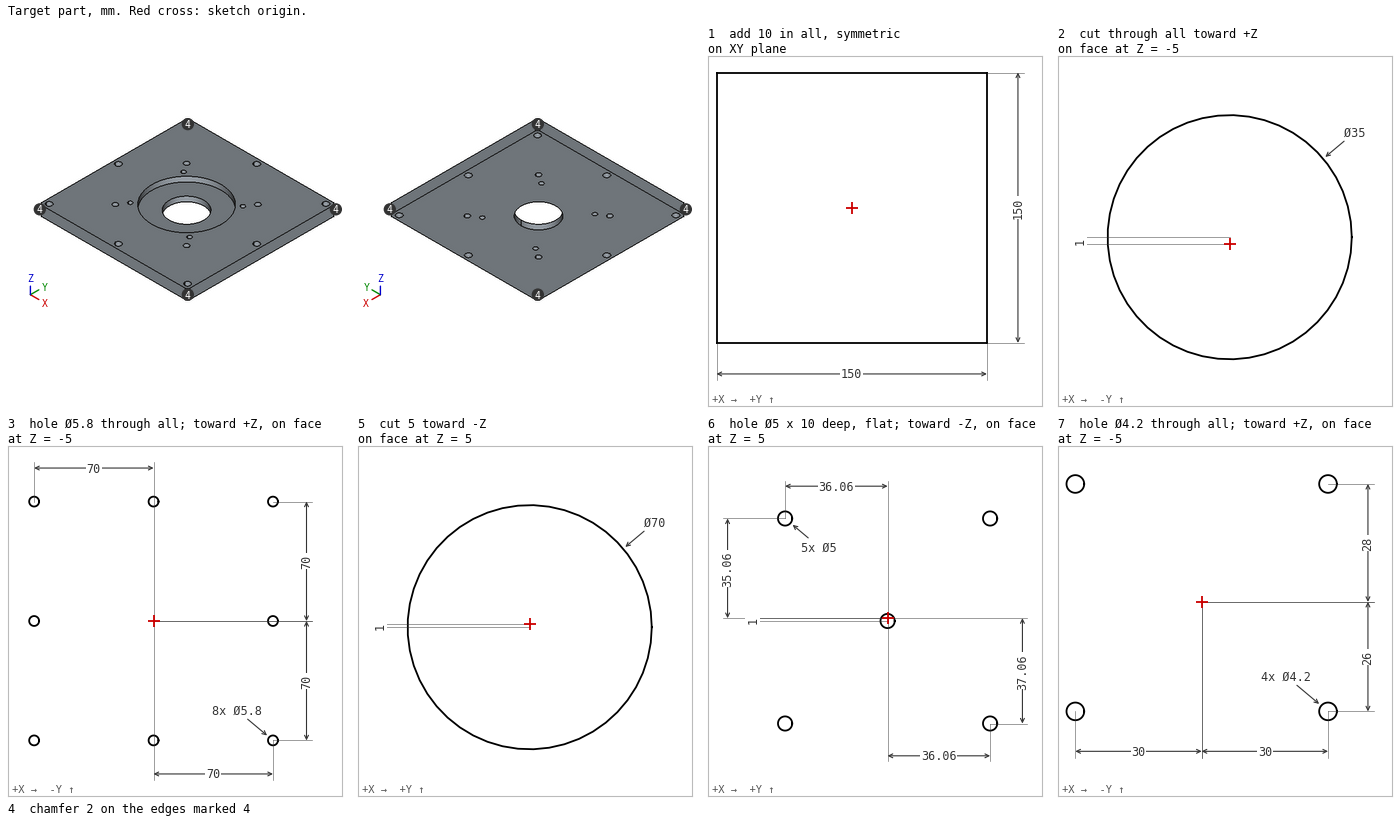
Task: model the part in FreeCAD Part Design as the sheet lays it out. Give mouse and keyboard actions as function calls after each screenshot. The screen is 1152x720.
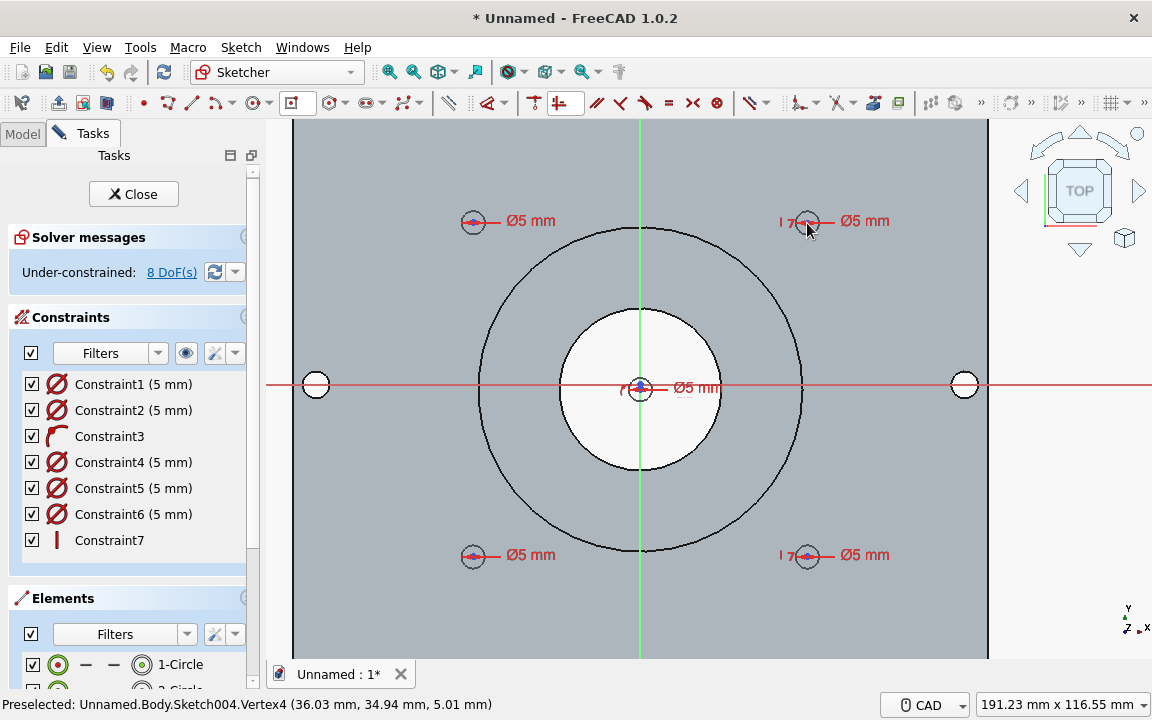
click(473, 223)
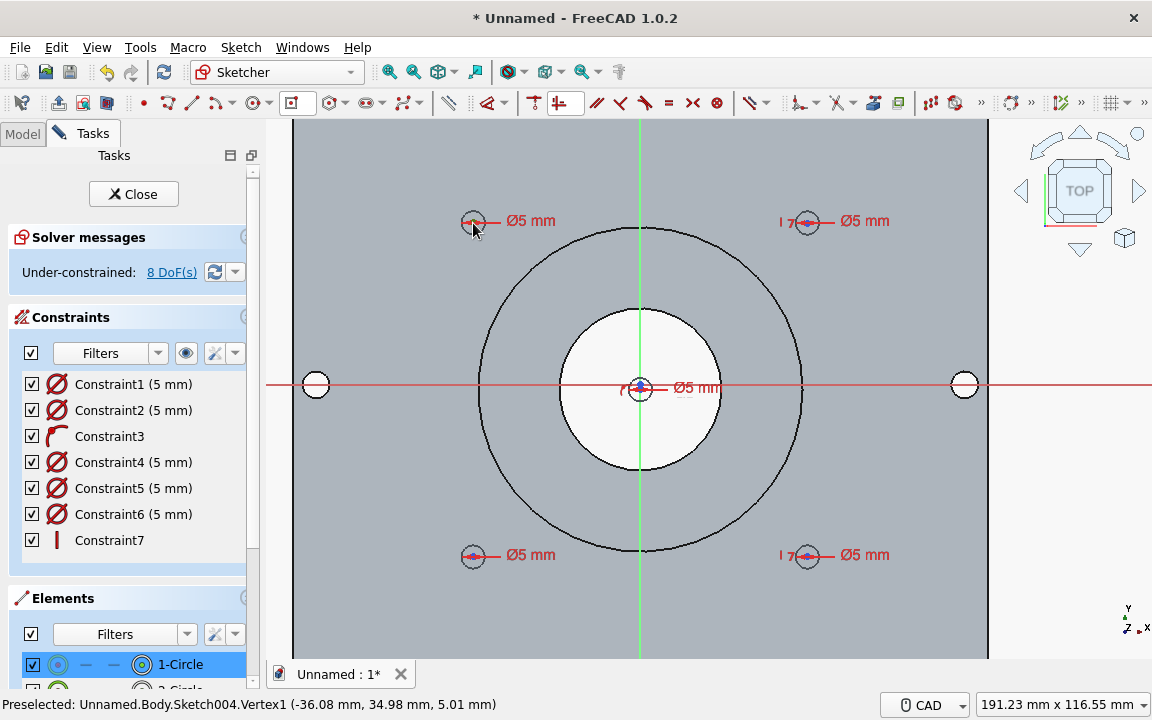
click(807, 223)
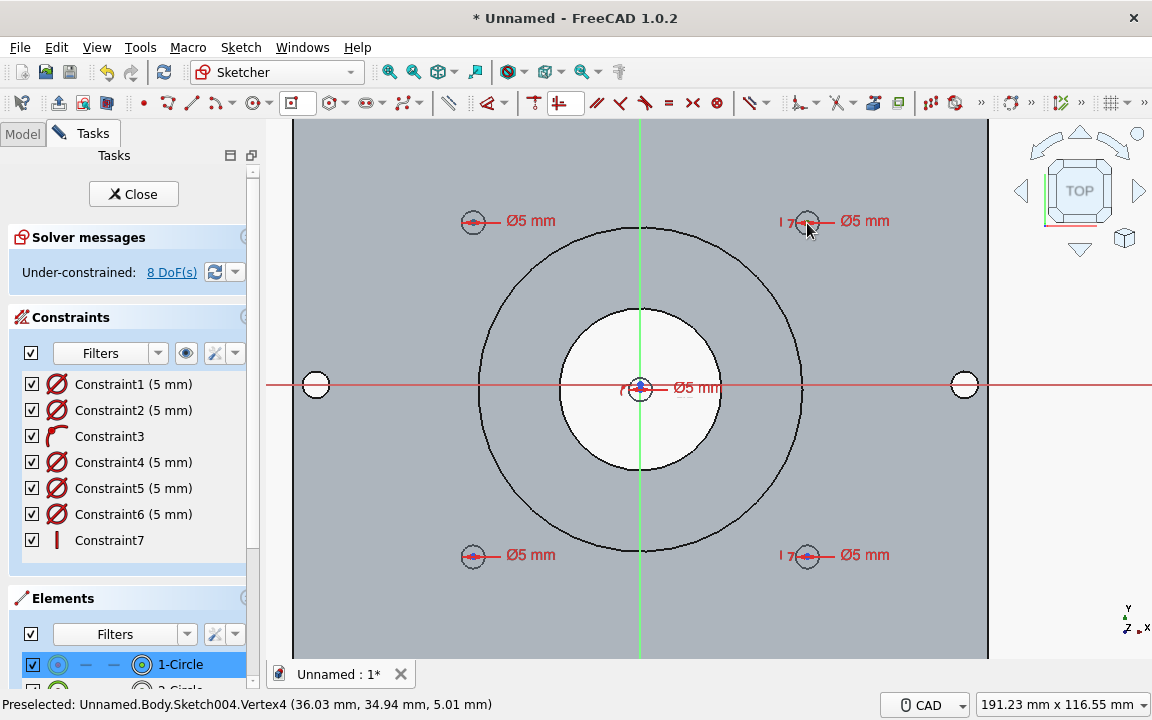
key(h)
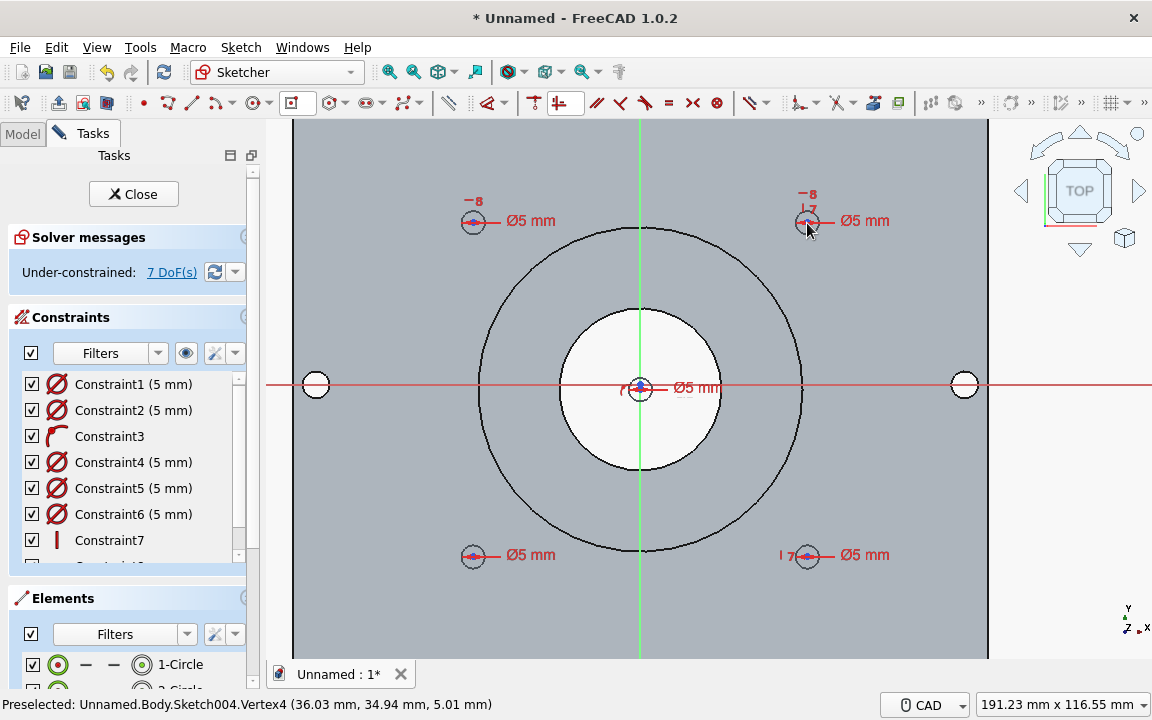
click(473, 223)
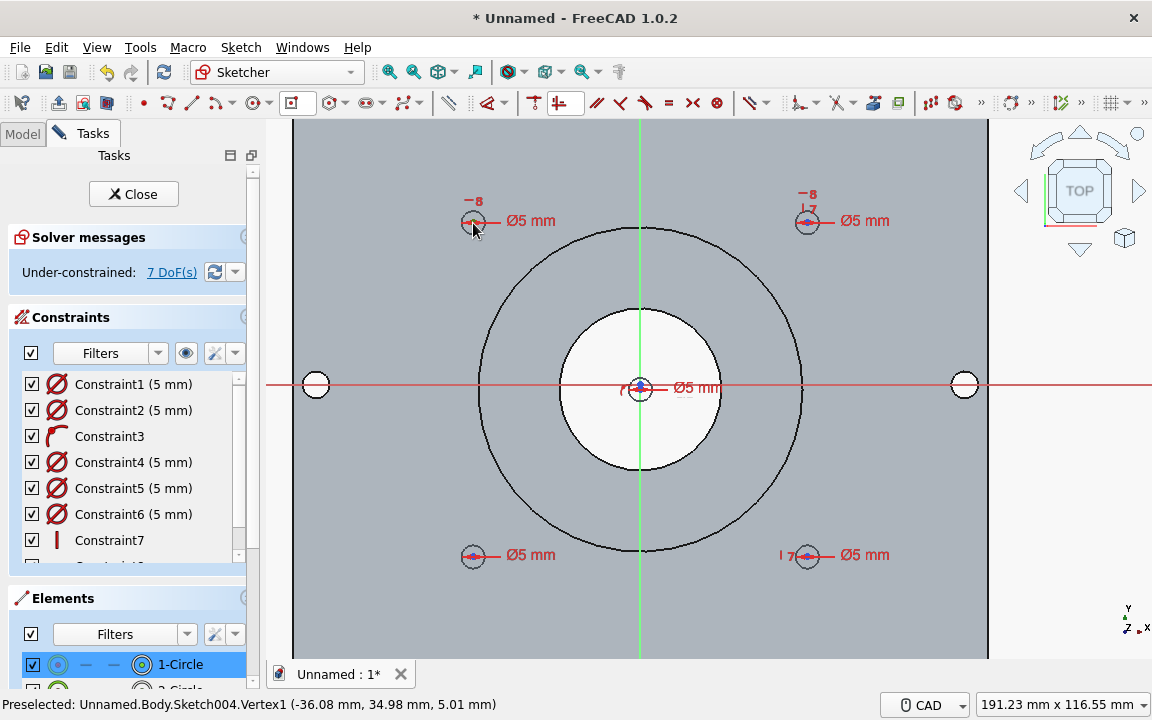
click(473, 557)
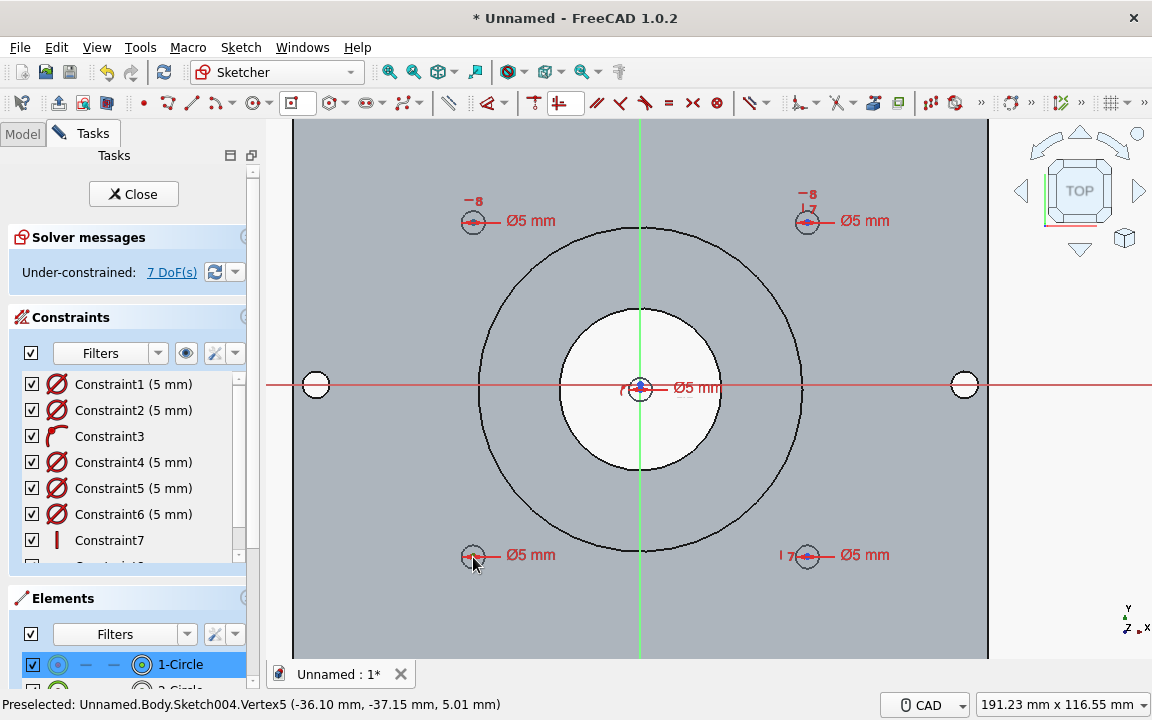
key(v)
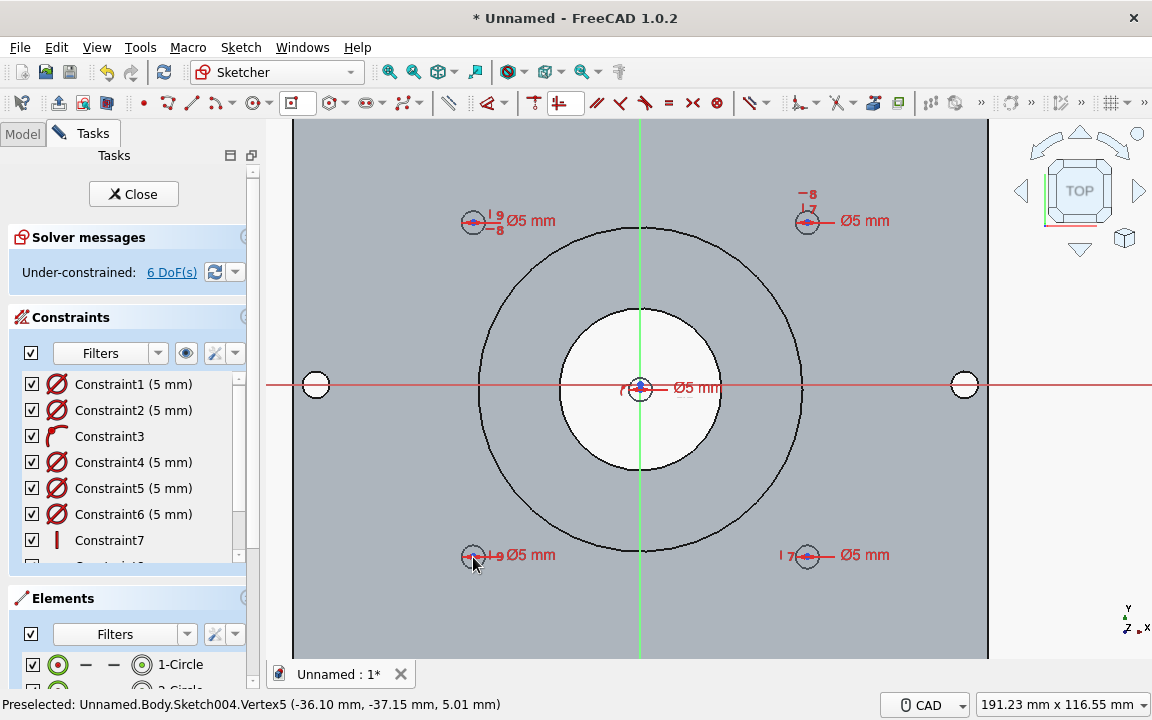
click(807, 557)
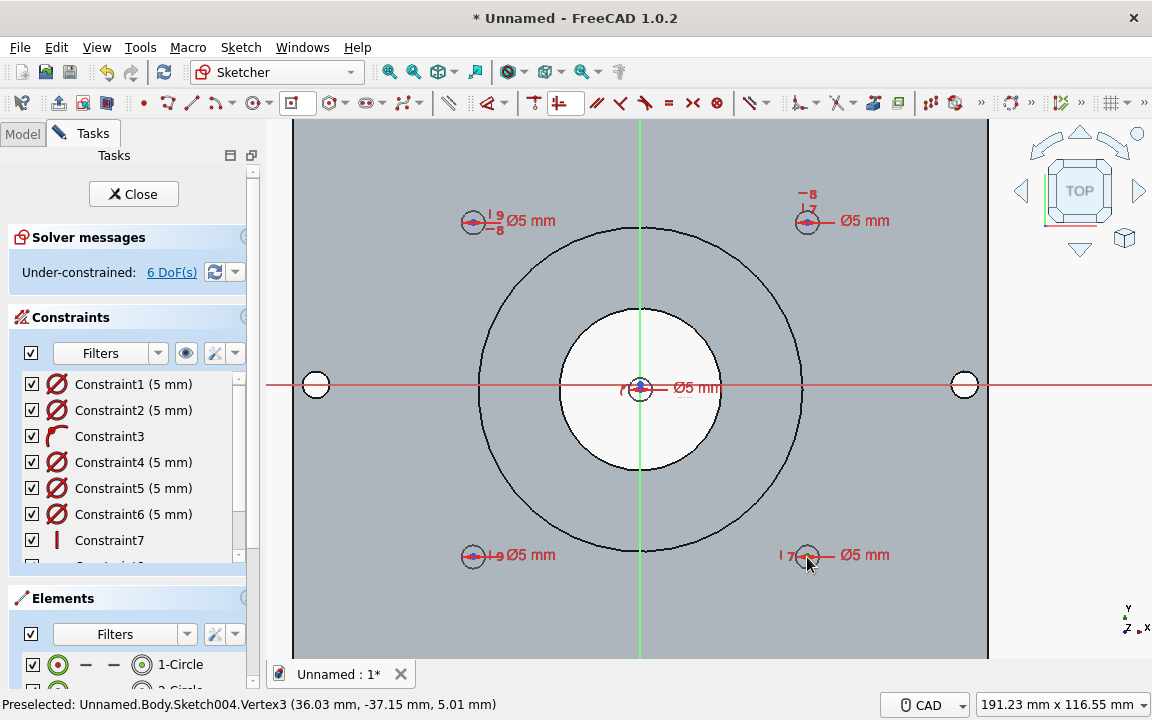
click(473, 557)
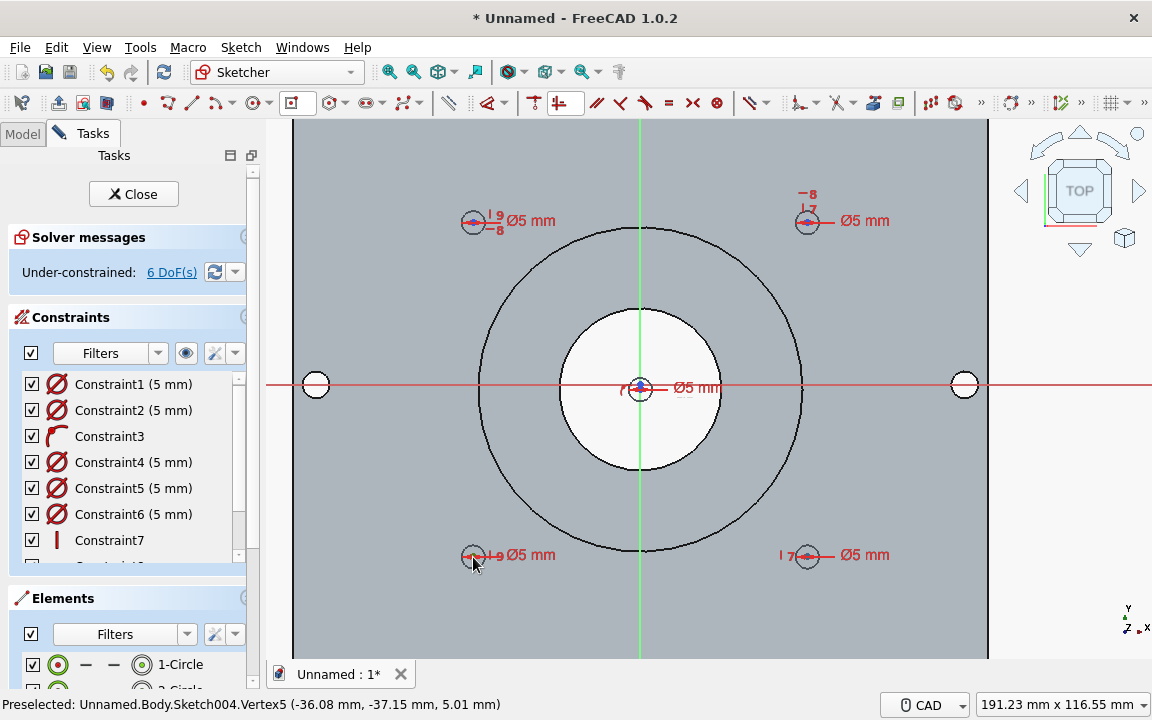
click(578, 104)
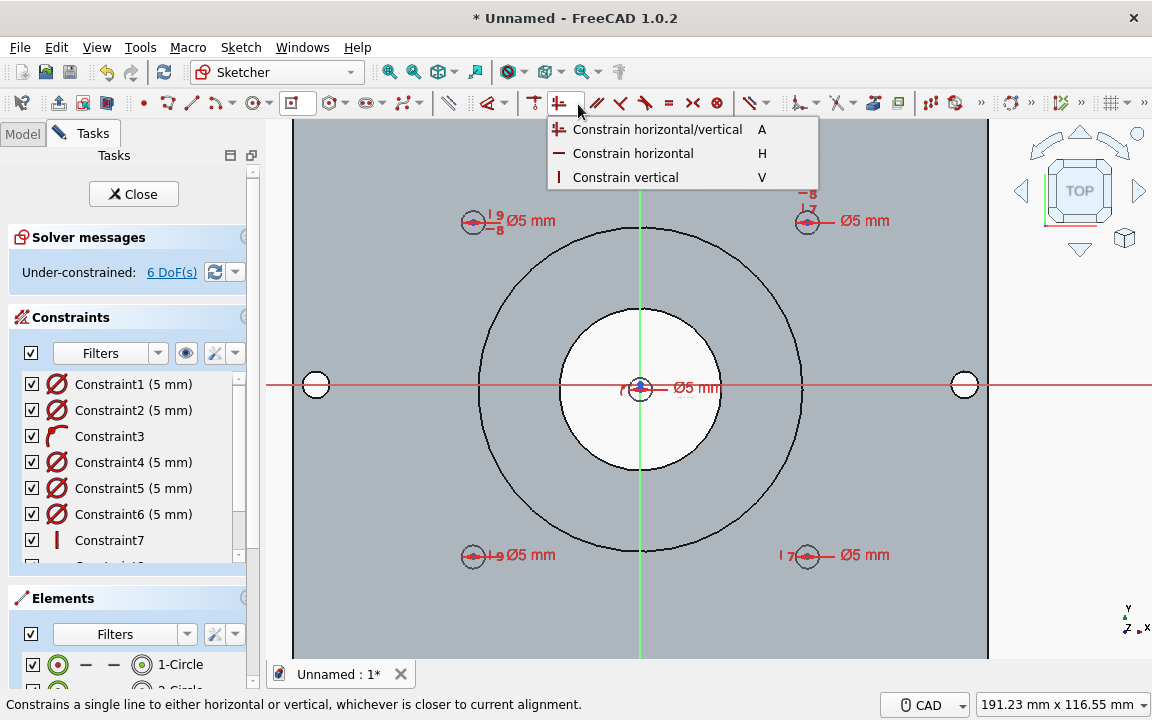
click(683, 153)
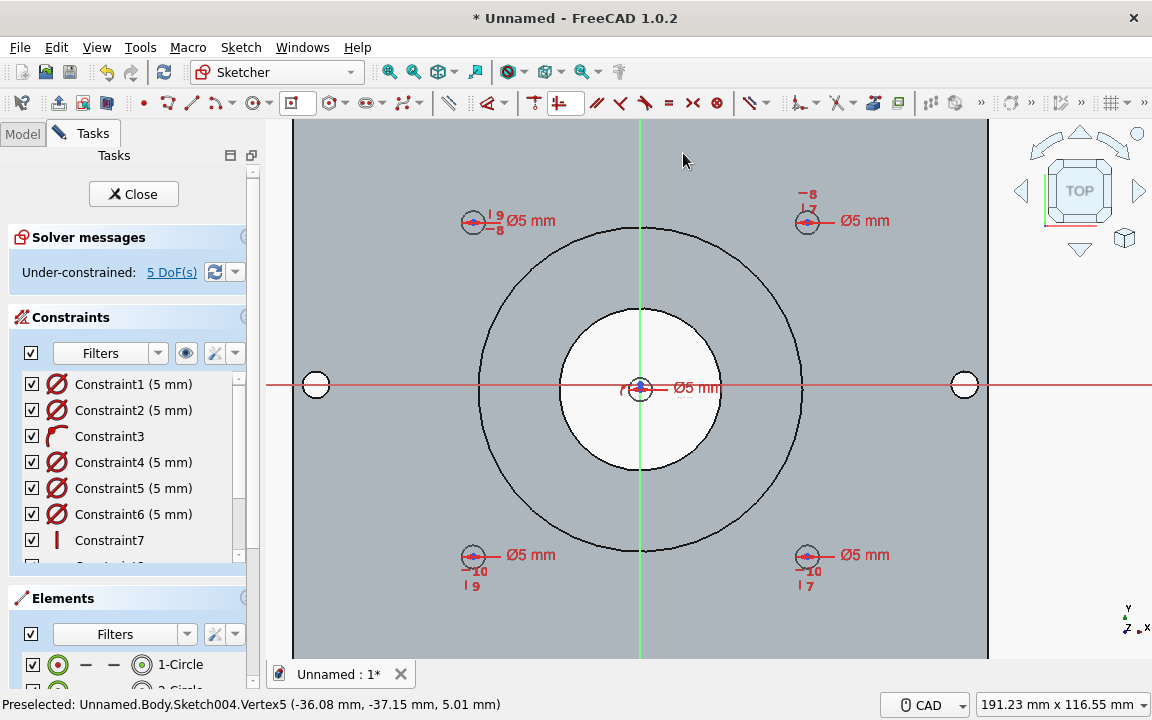
key(d)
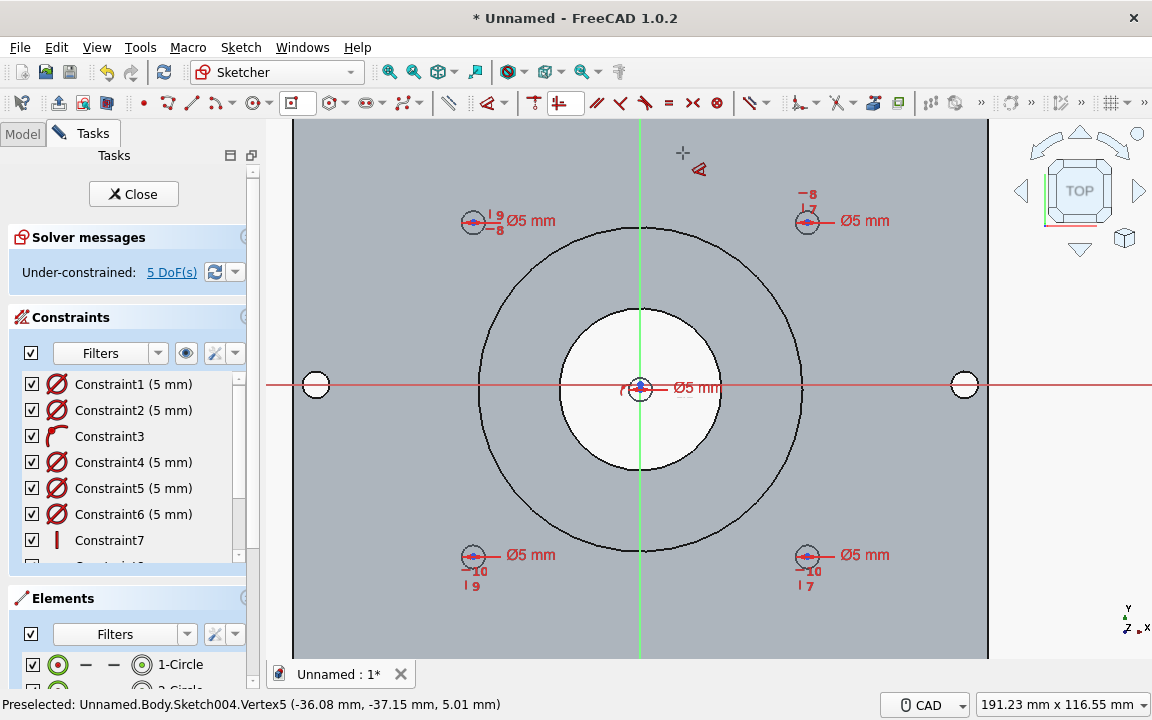
scroll(640, 390, up, 11)